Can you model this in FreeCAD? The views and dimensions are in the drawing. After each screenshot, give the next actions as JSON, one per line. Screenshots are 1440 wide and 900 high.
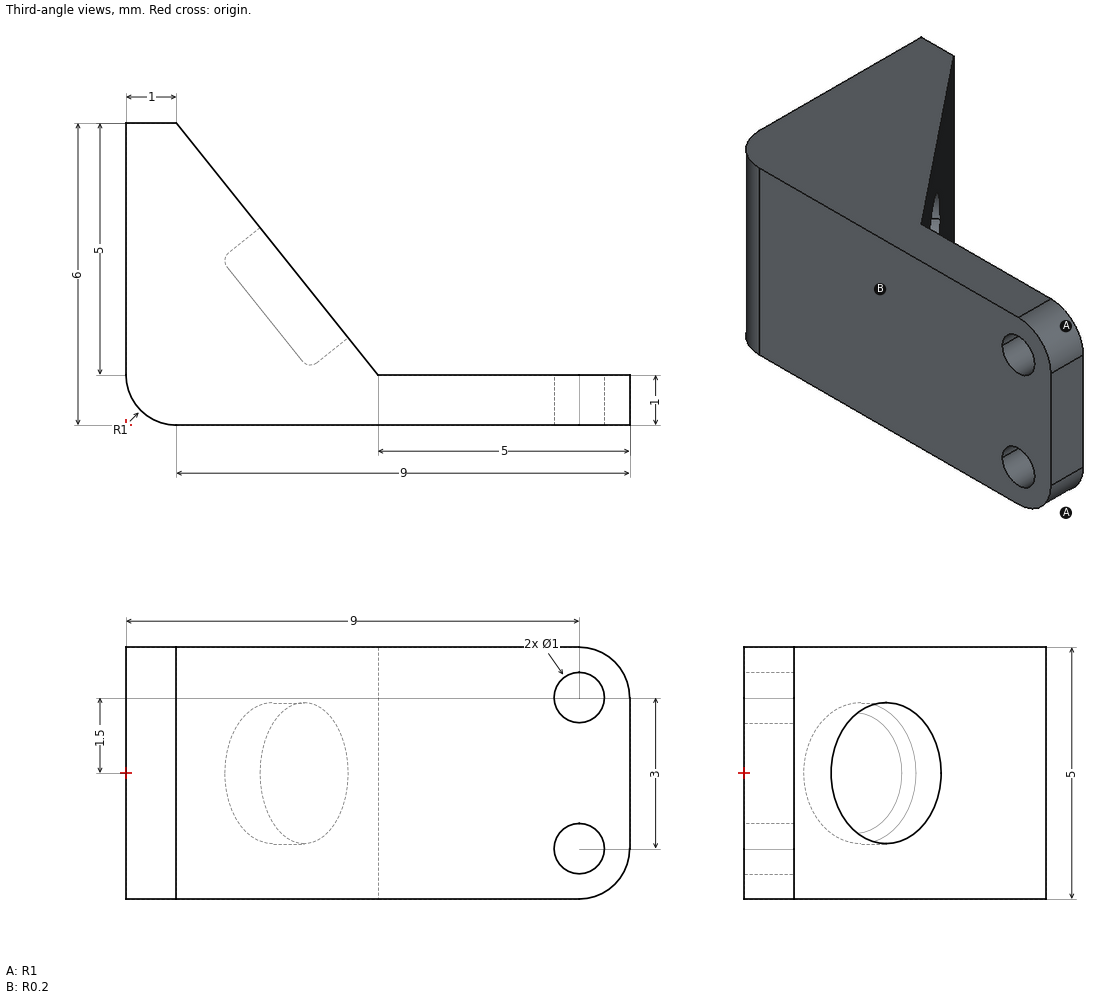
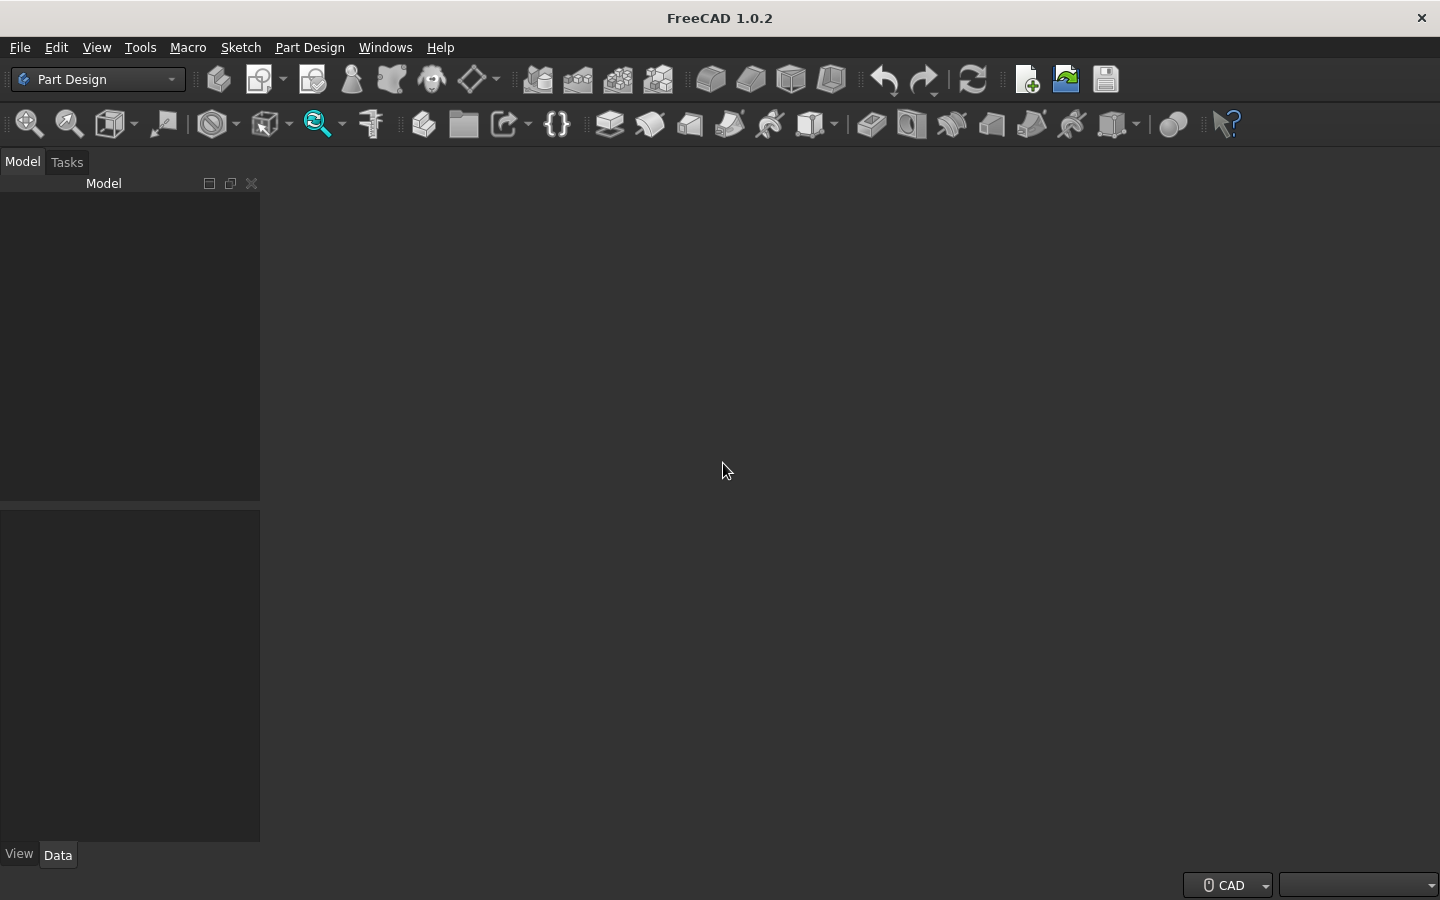
{"action": "left_click", "coordinate": [1026, 80]}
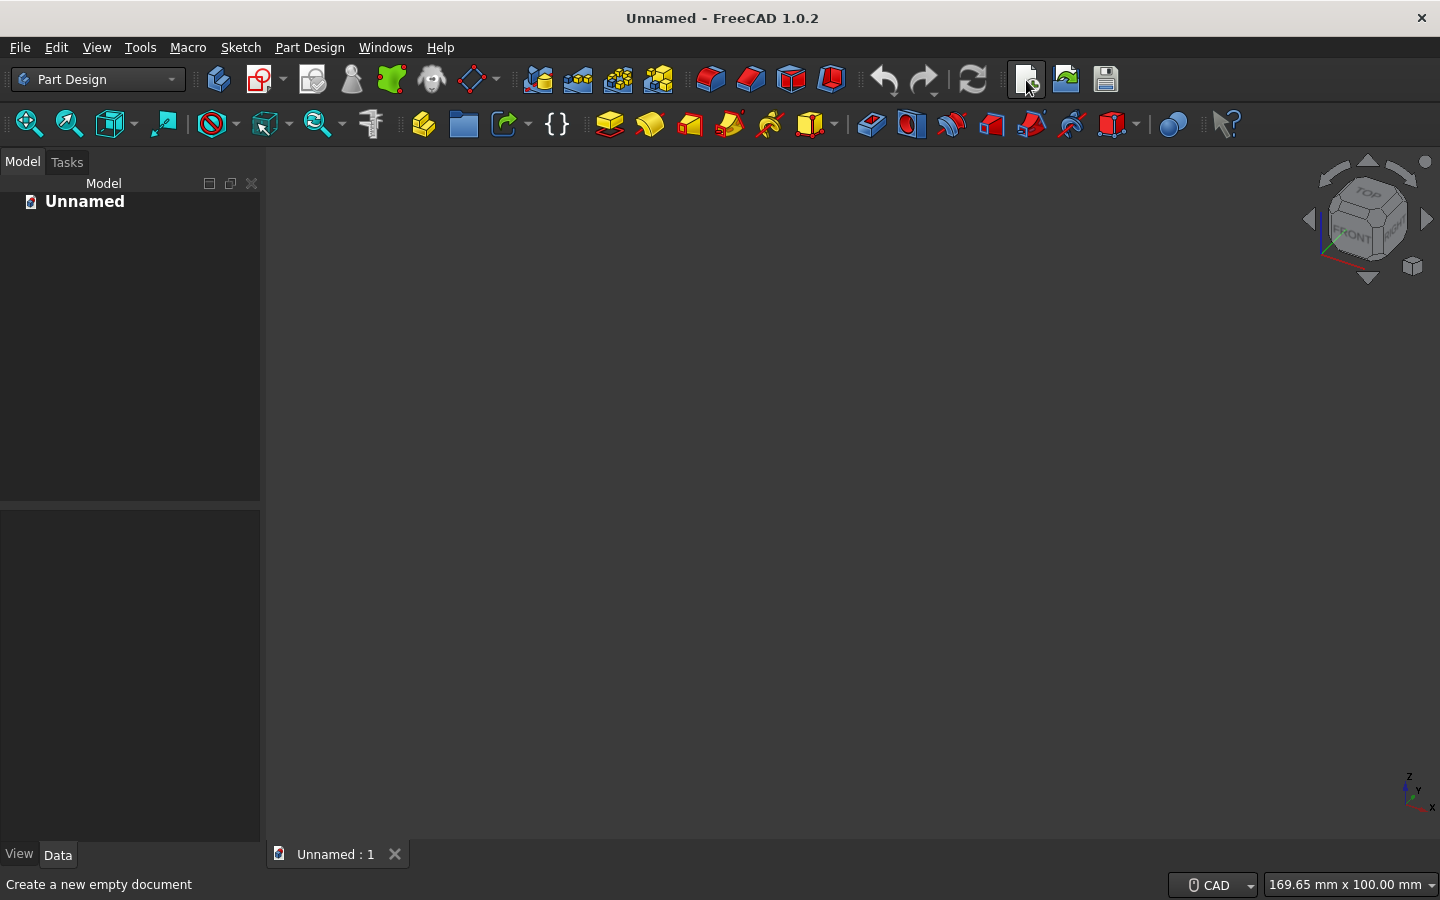
{"action": "left_click", "coordinate": [260, 80]}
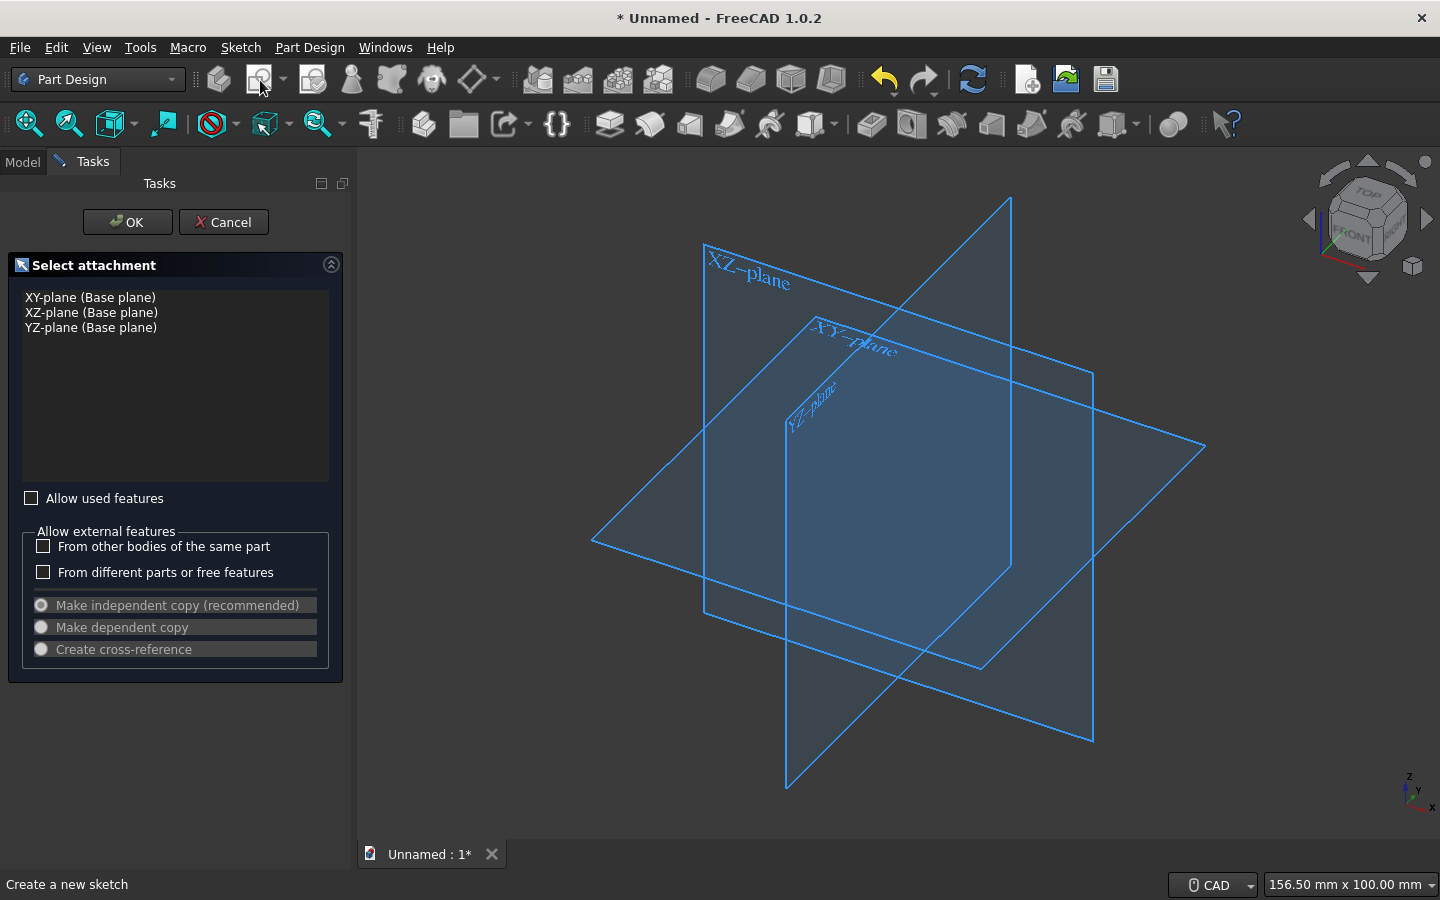
{"action": "left_click", "coordinate": [82, 298]}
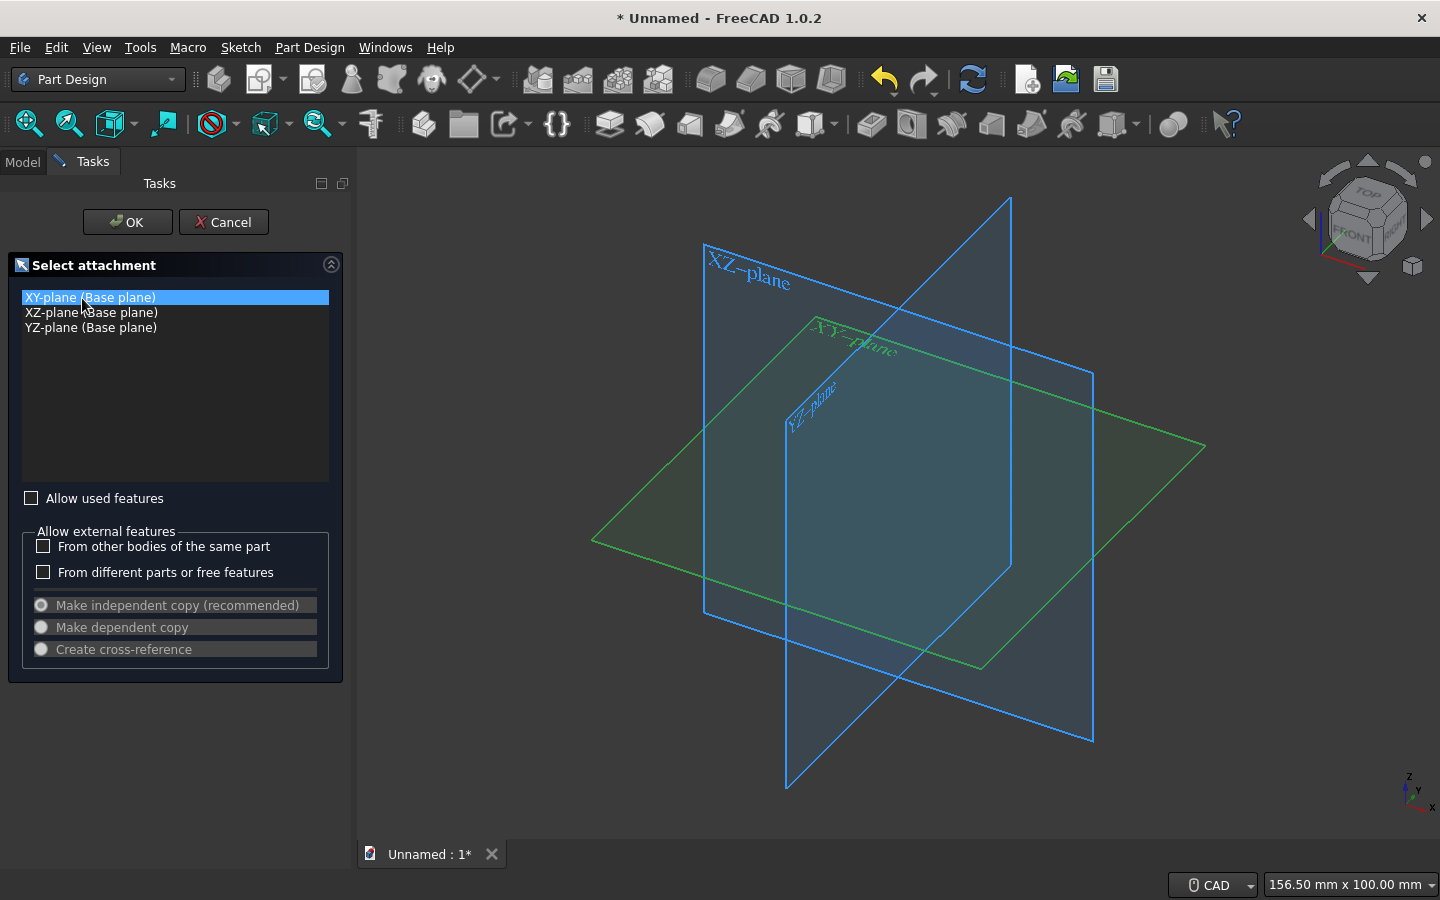
{"action": "left_click", "coordinate": [128, 222]}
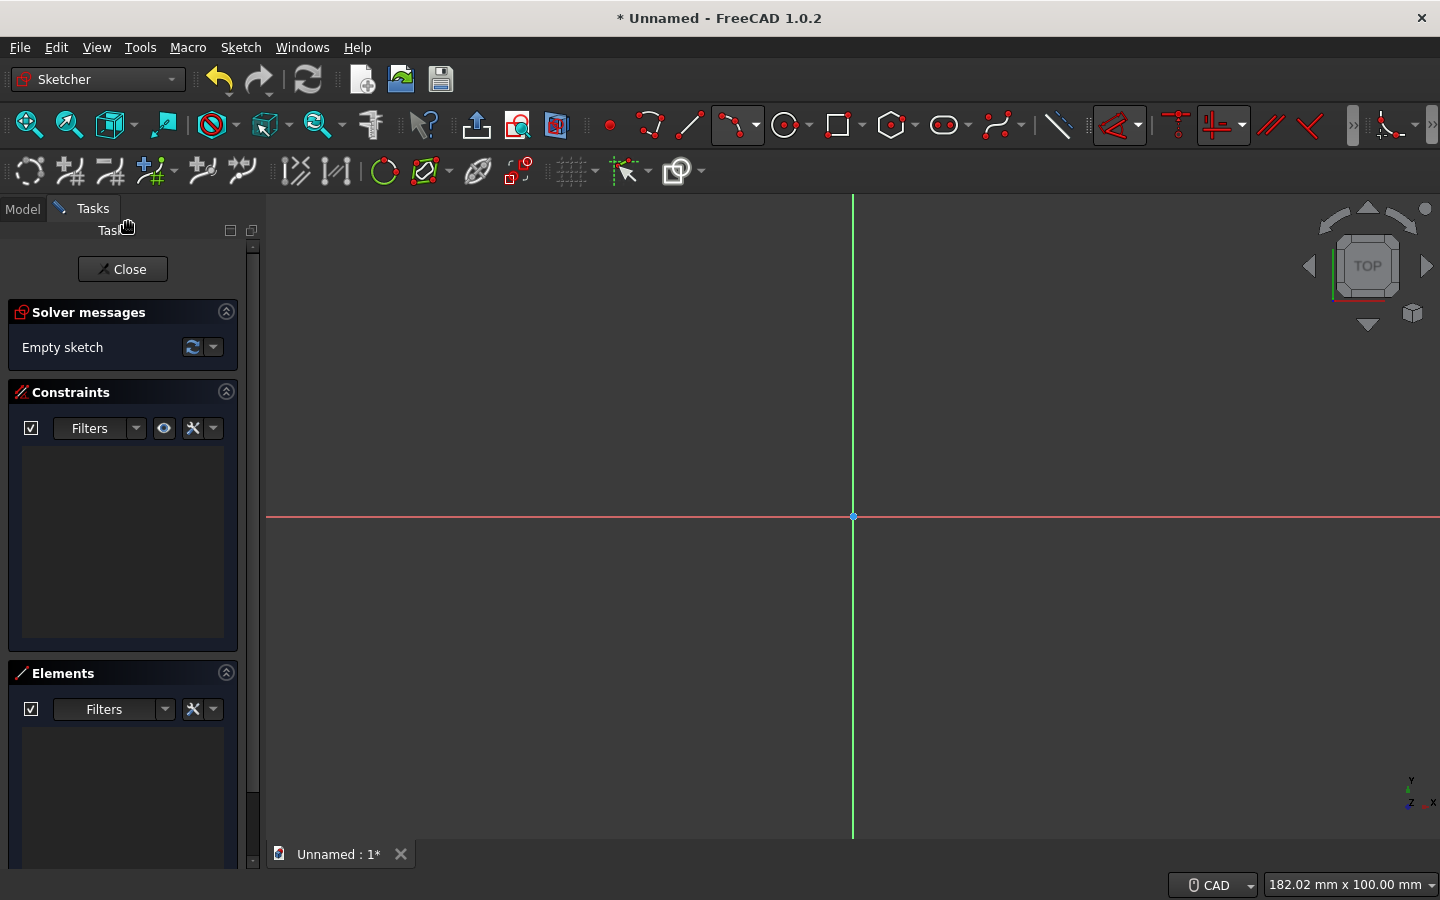
{"action": "scroll", "coordinate": [895, 495], "scroll_direction": "up", "scroll_amount": 12}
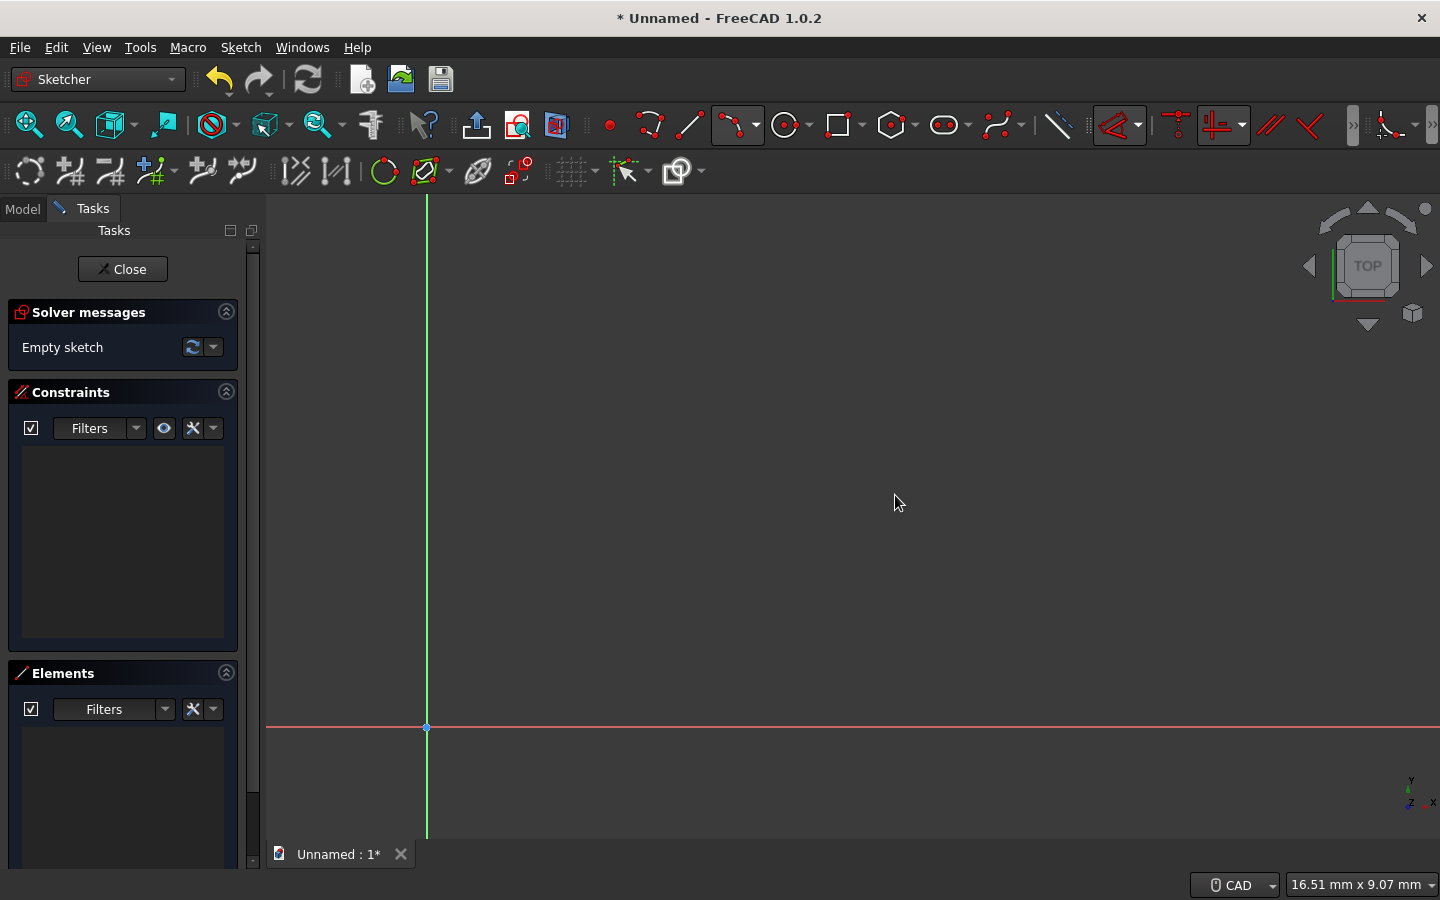
{"action": "left_click", "coordinate": [650, 126]}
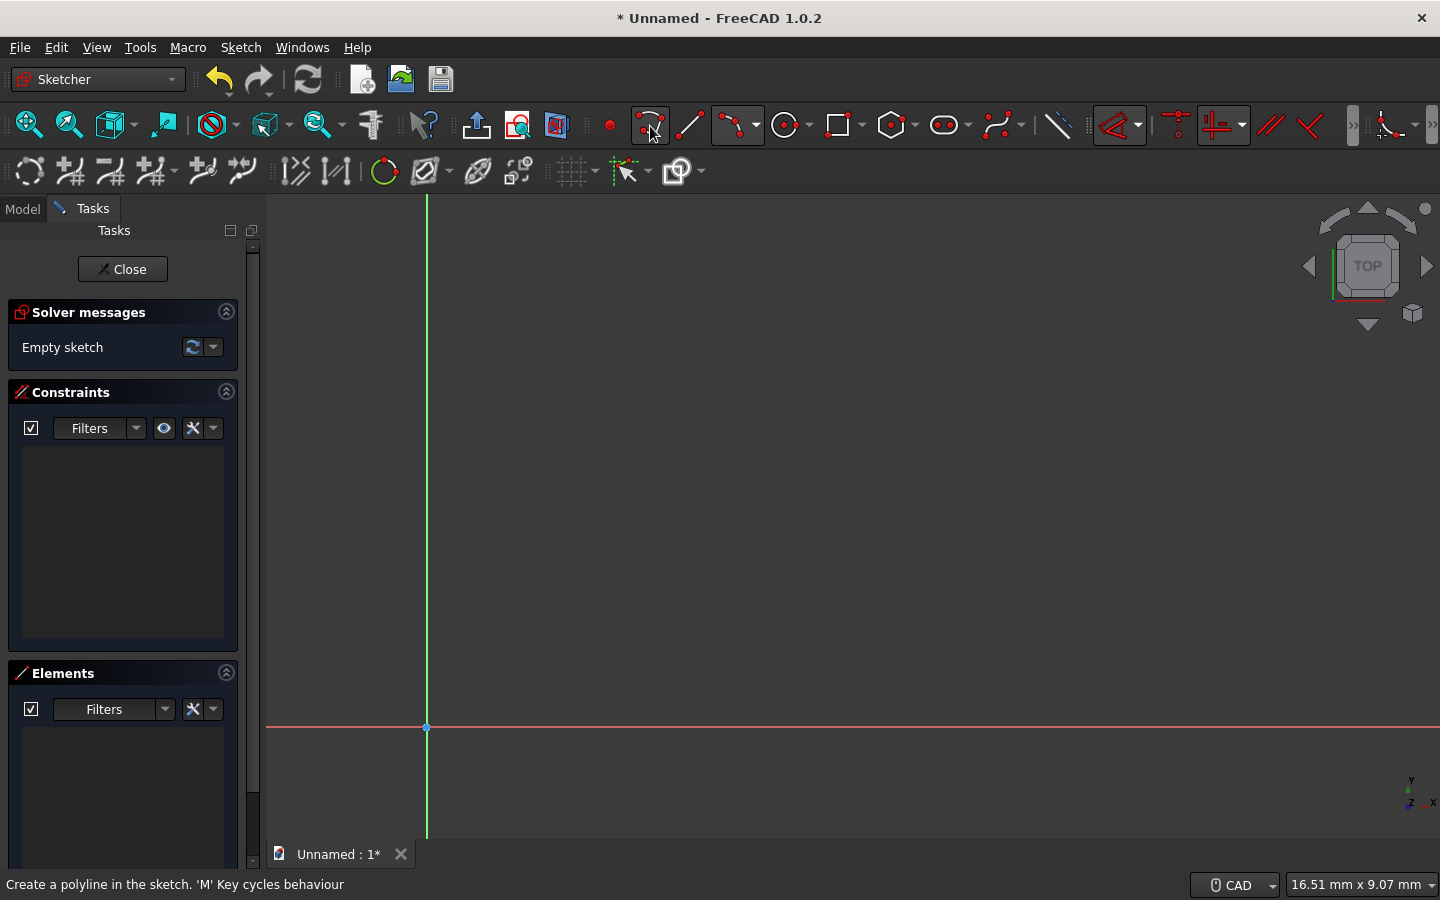
{"action": "left_click", "coordinate": [498, 727]}
{"action": "left_click", "coordinate": [1138, 718]}
{"action": "left_click", "coordinate": [1138, 656]}
{"action": "left_click", "coordinate": [782, 656]}
{"action": "left_click", "coordinate": [498, 301]}
{"action": "left_click", "coordinate": [427, 301]}
{"action": "left_click", "coordinate": [436, 656]}
{"action": "right_click", "coordinate": [436, 656]}